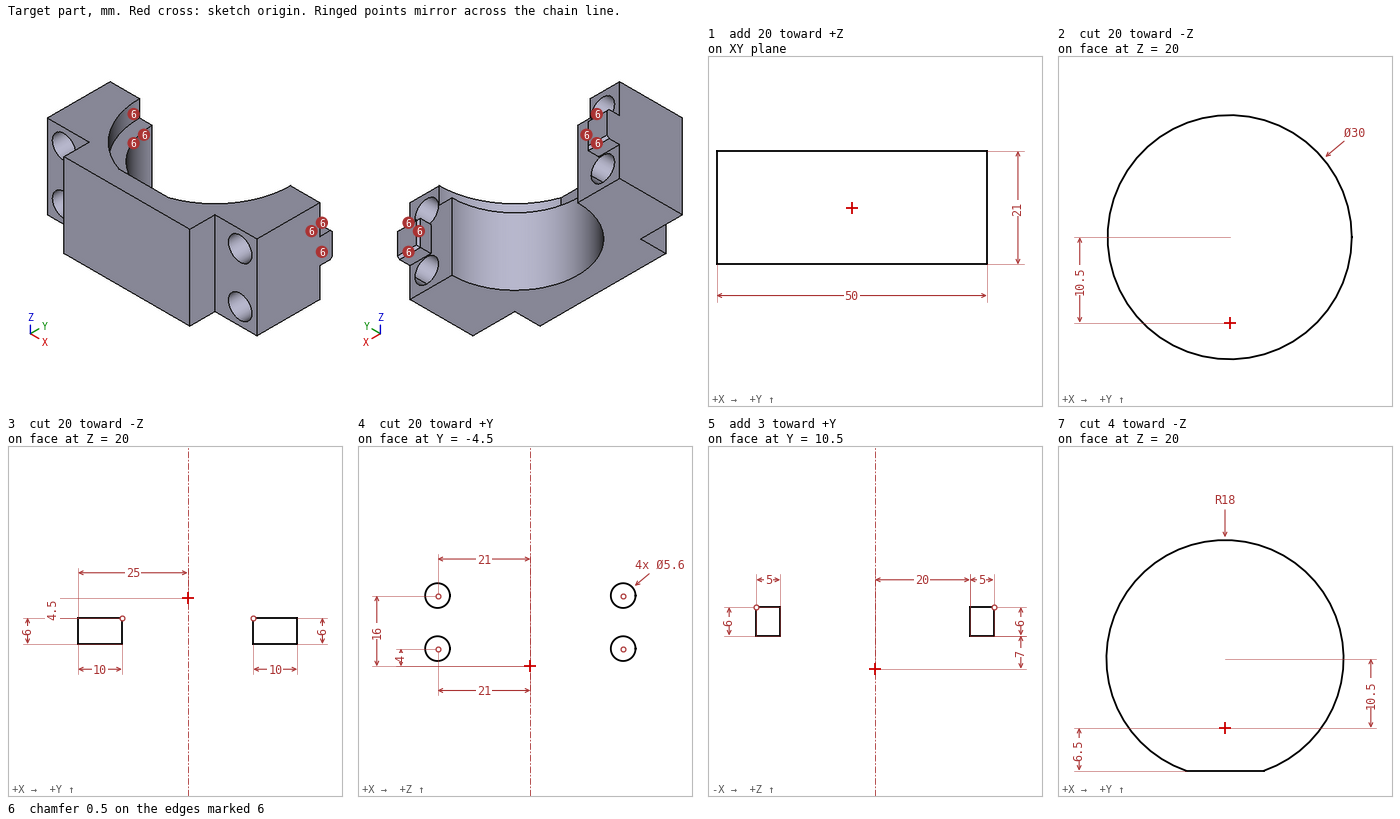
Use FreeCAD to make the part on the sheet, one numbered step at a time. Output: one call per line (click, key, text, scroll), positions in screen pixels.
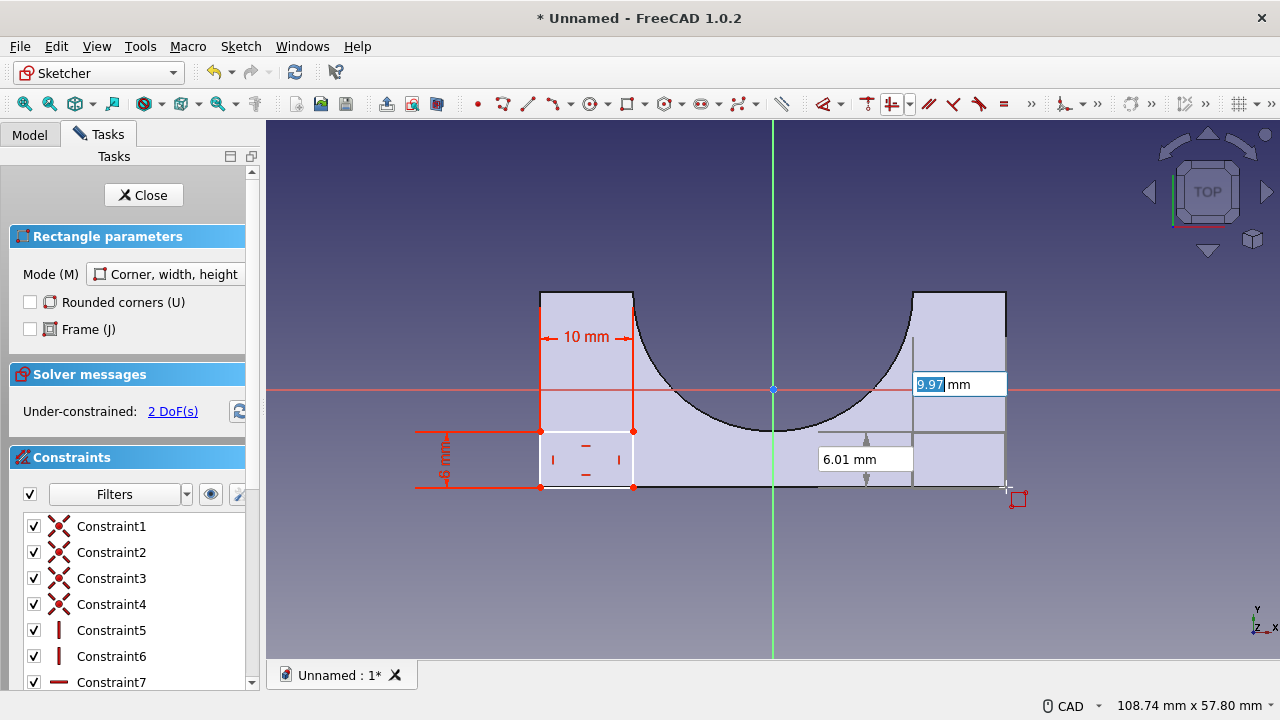
text(10)
key(Tab)
text(6)
key(Return)
key(Escape)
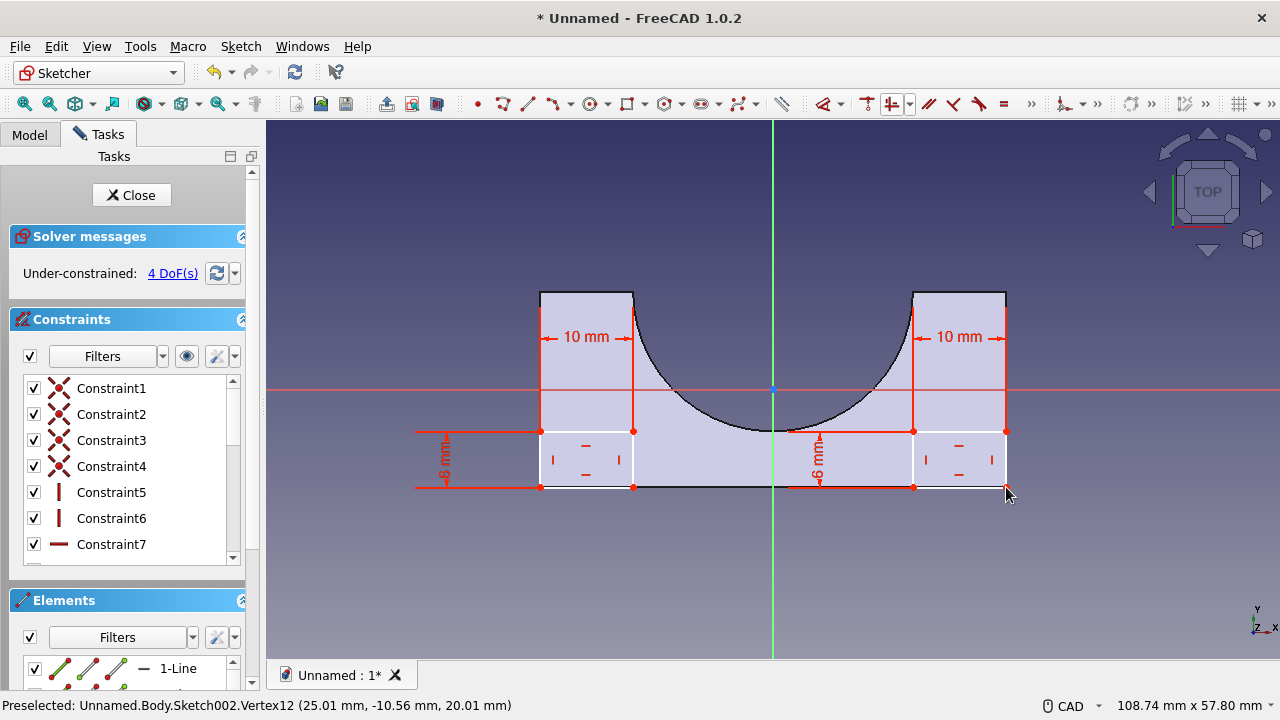
click(633, 432)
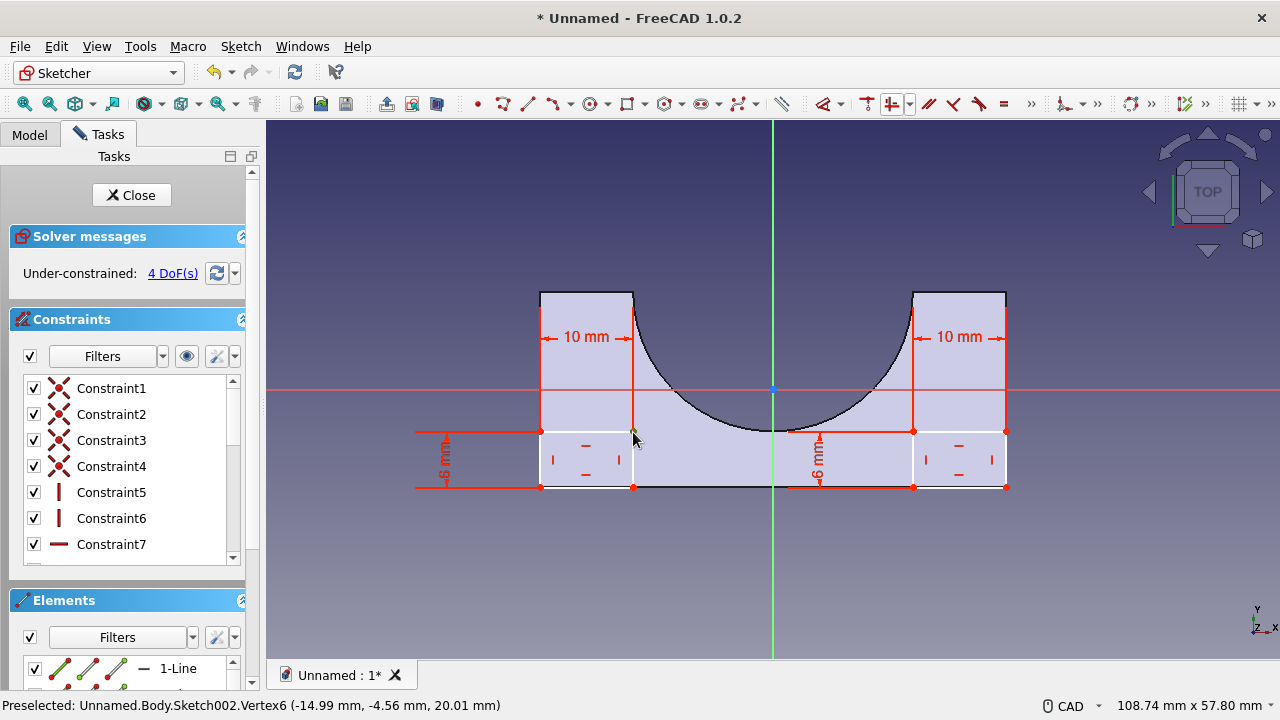
click(913, 432)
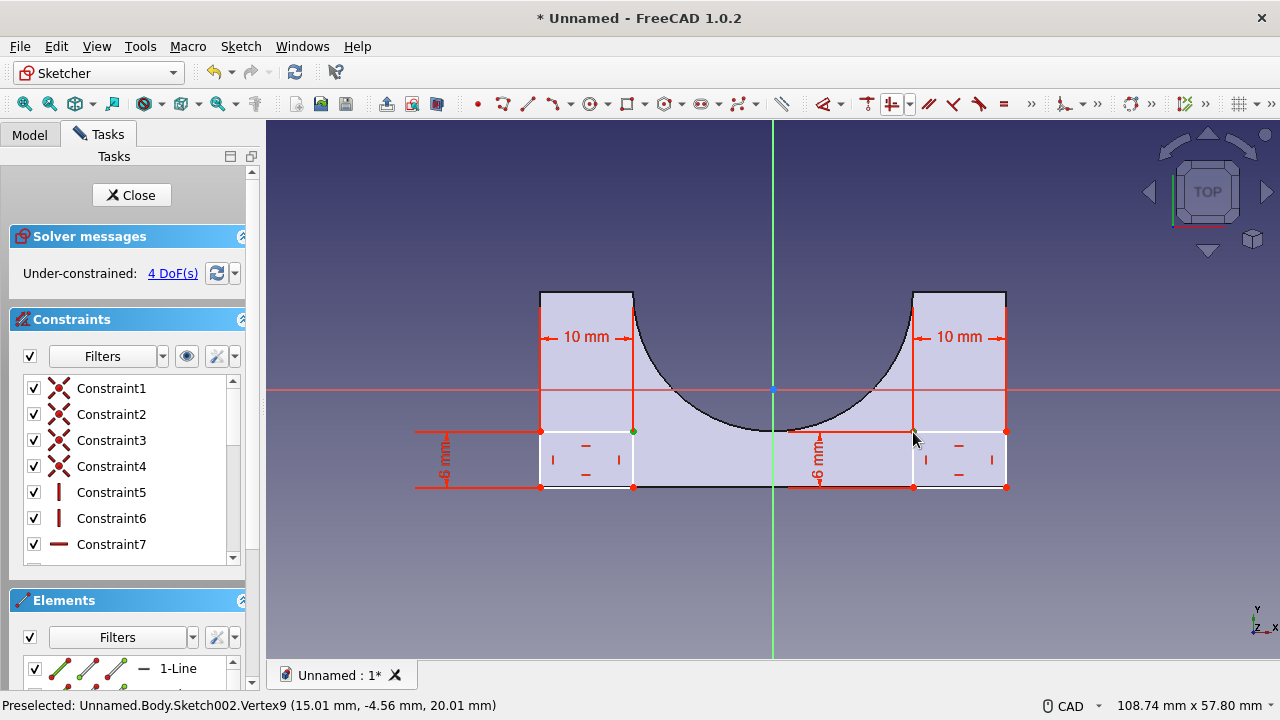
click(773, 596)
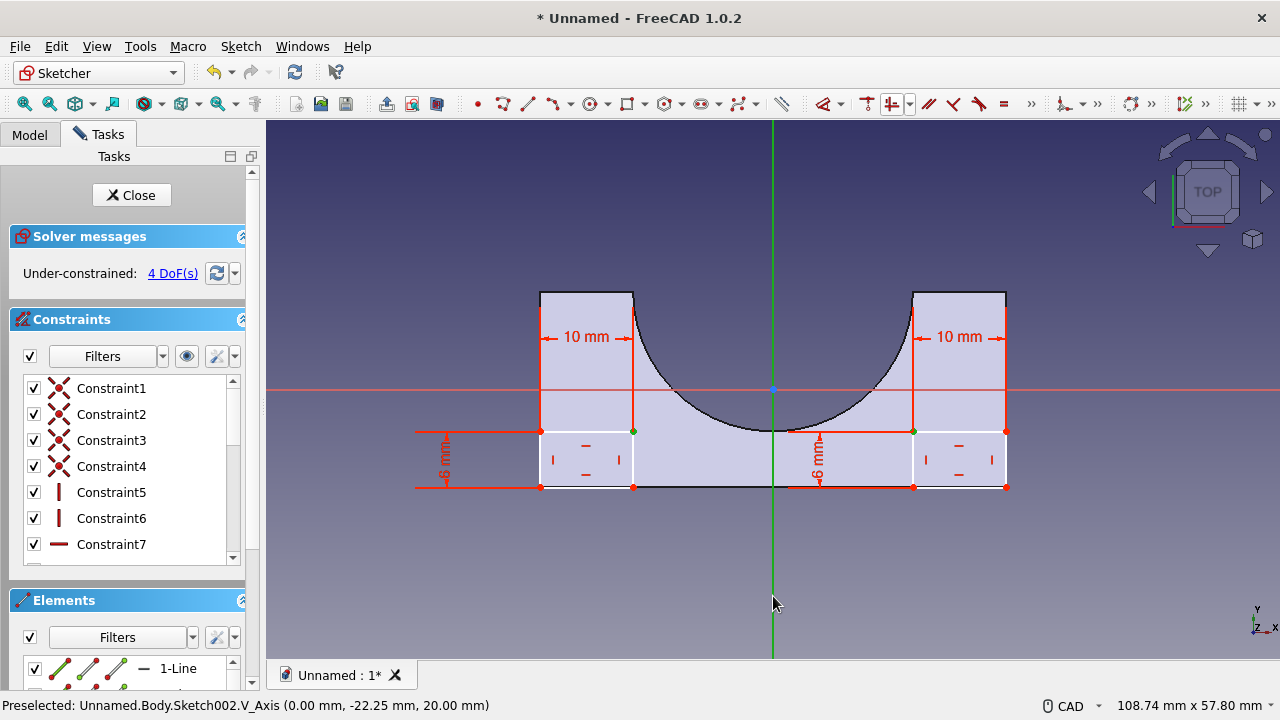
key(s)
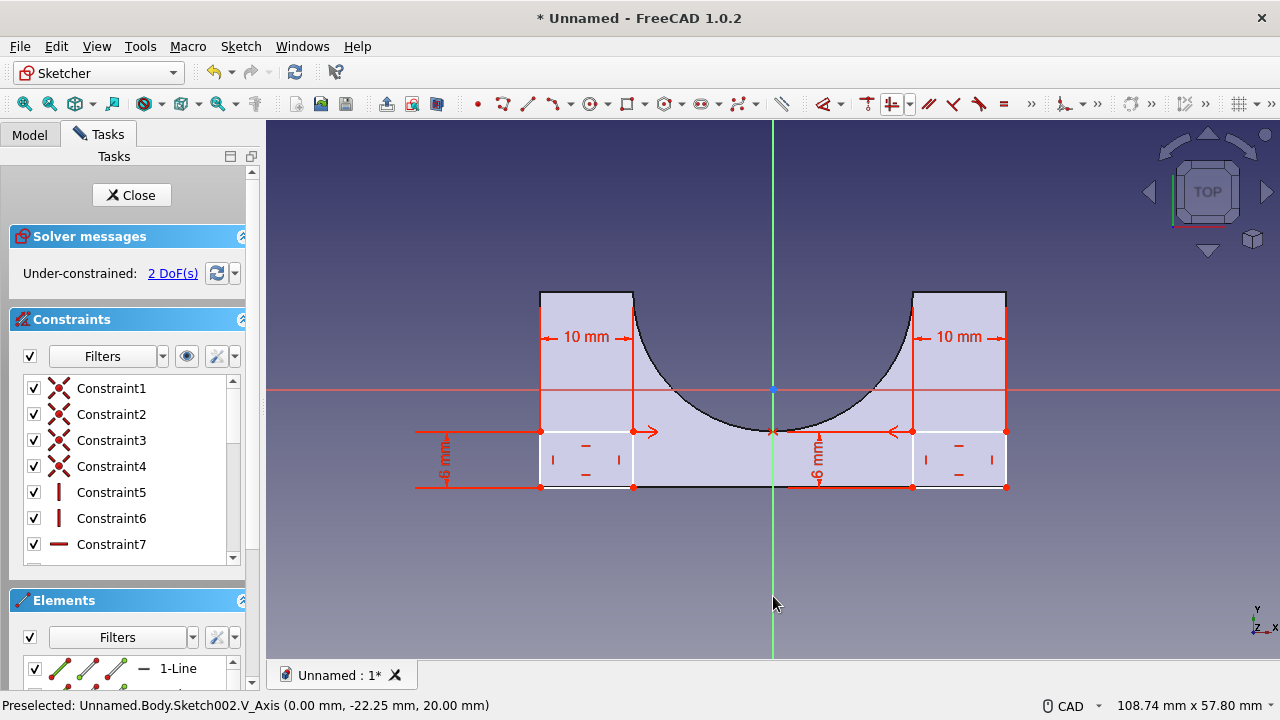
click(822, 104)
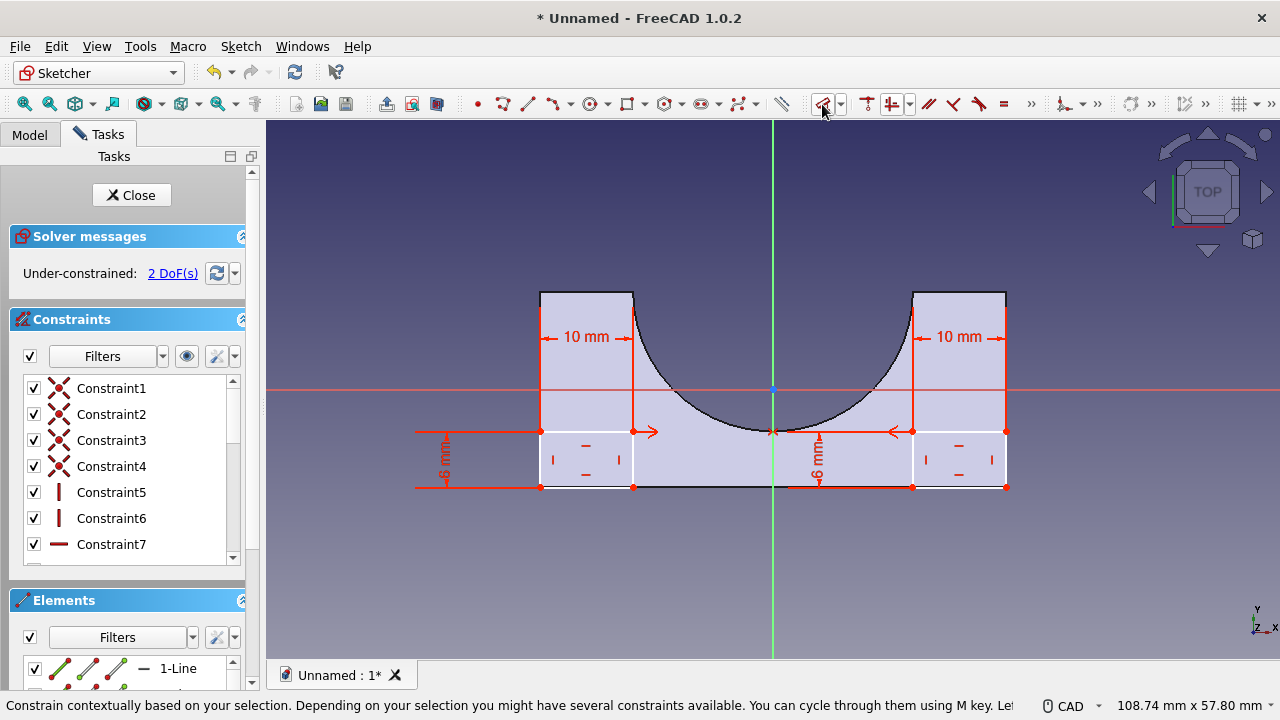
click(540, 432)
click(657, 356)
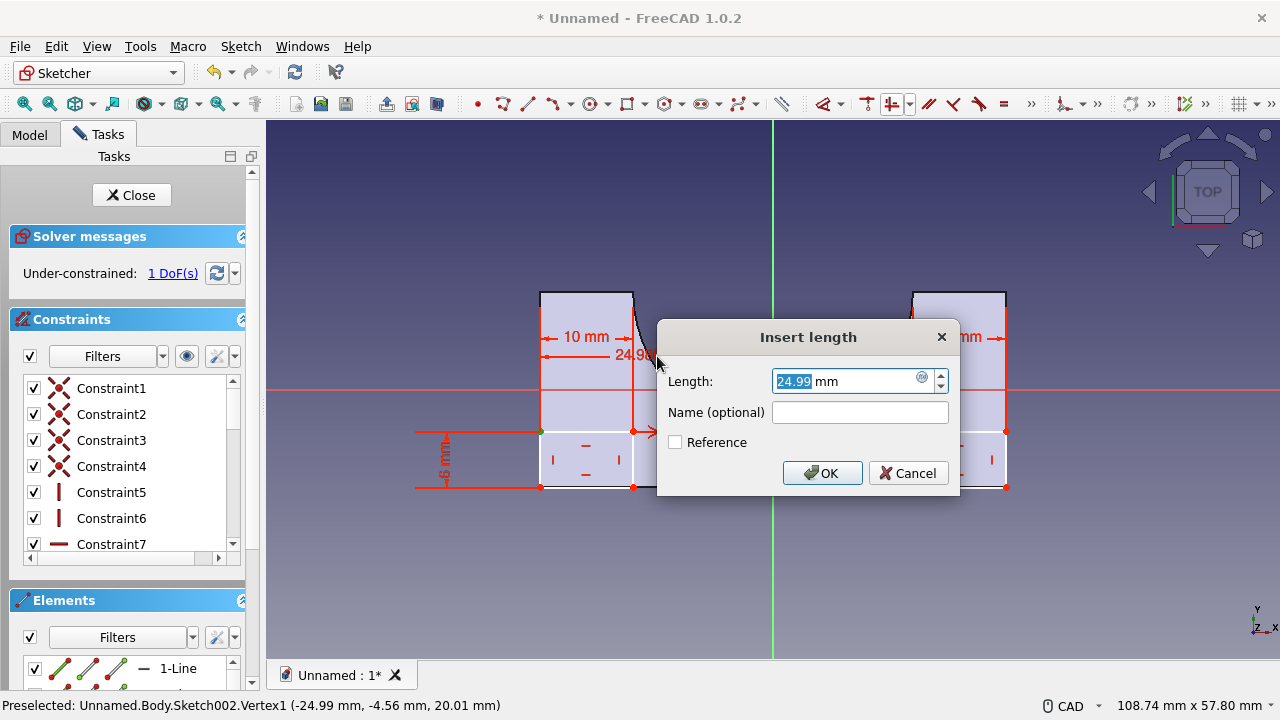
text(25)
key(Return)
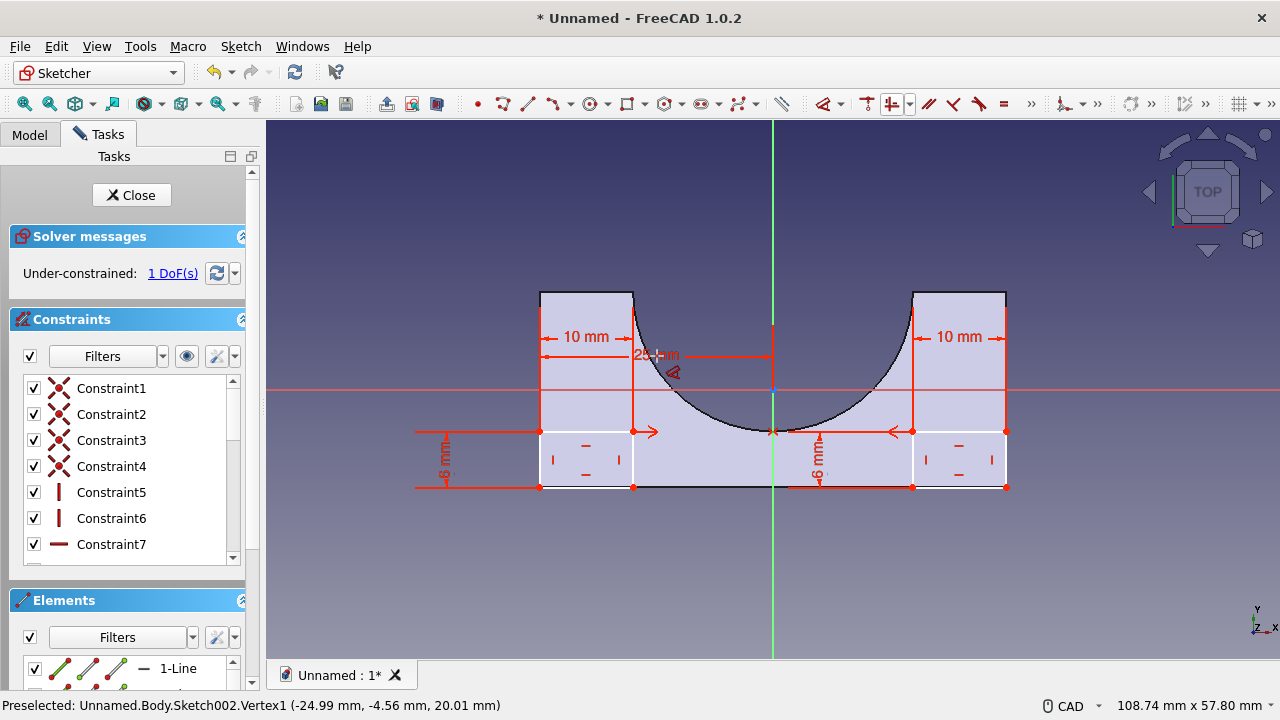
click(540, 432)
click(506, 411)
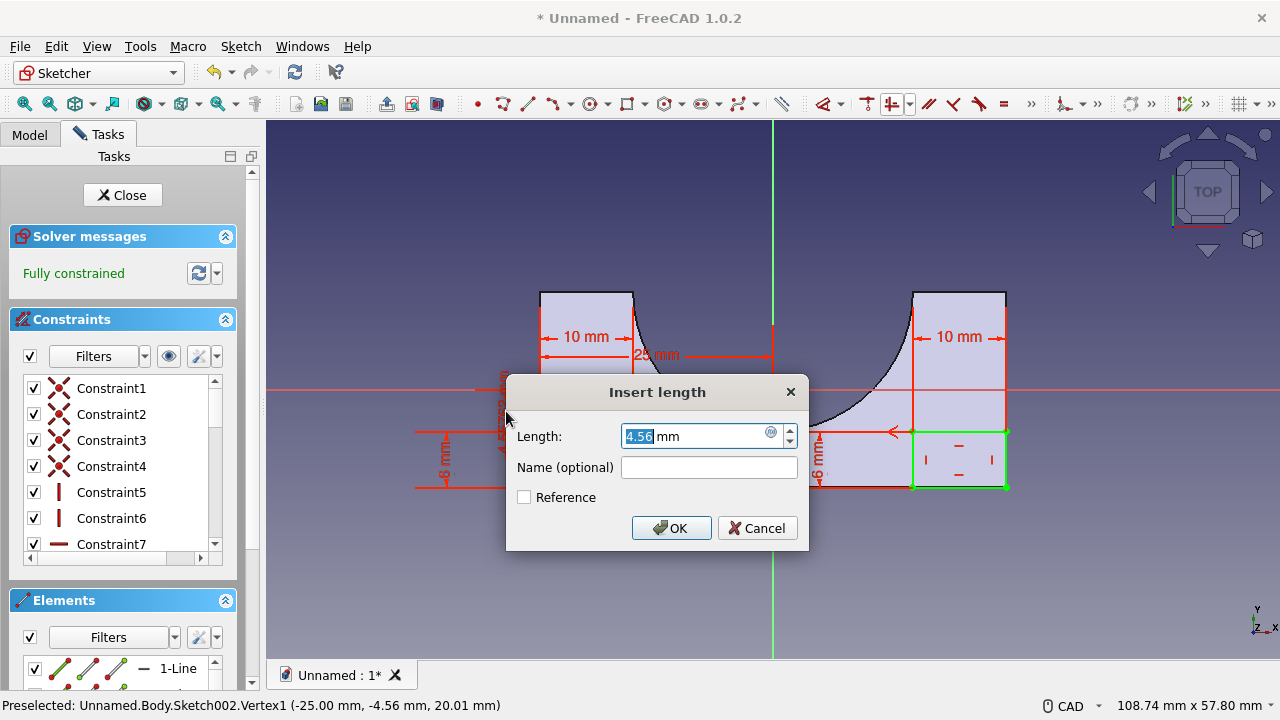
text(4.5)
key(Return)
key(Escape)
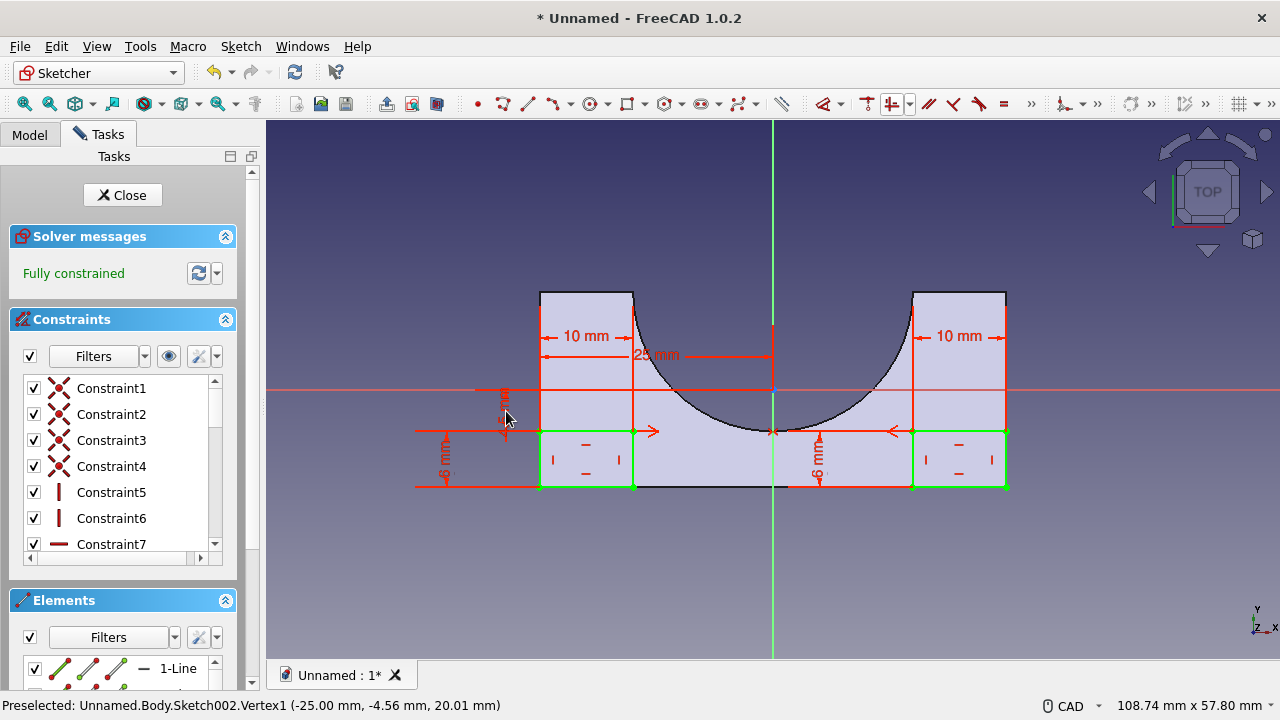
click(123, 195)